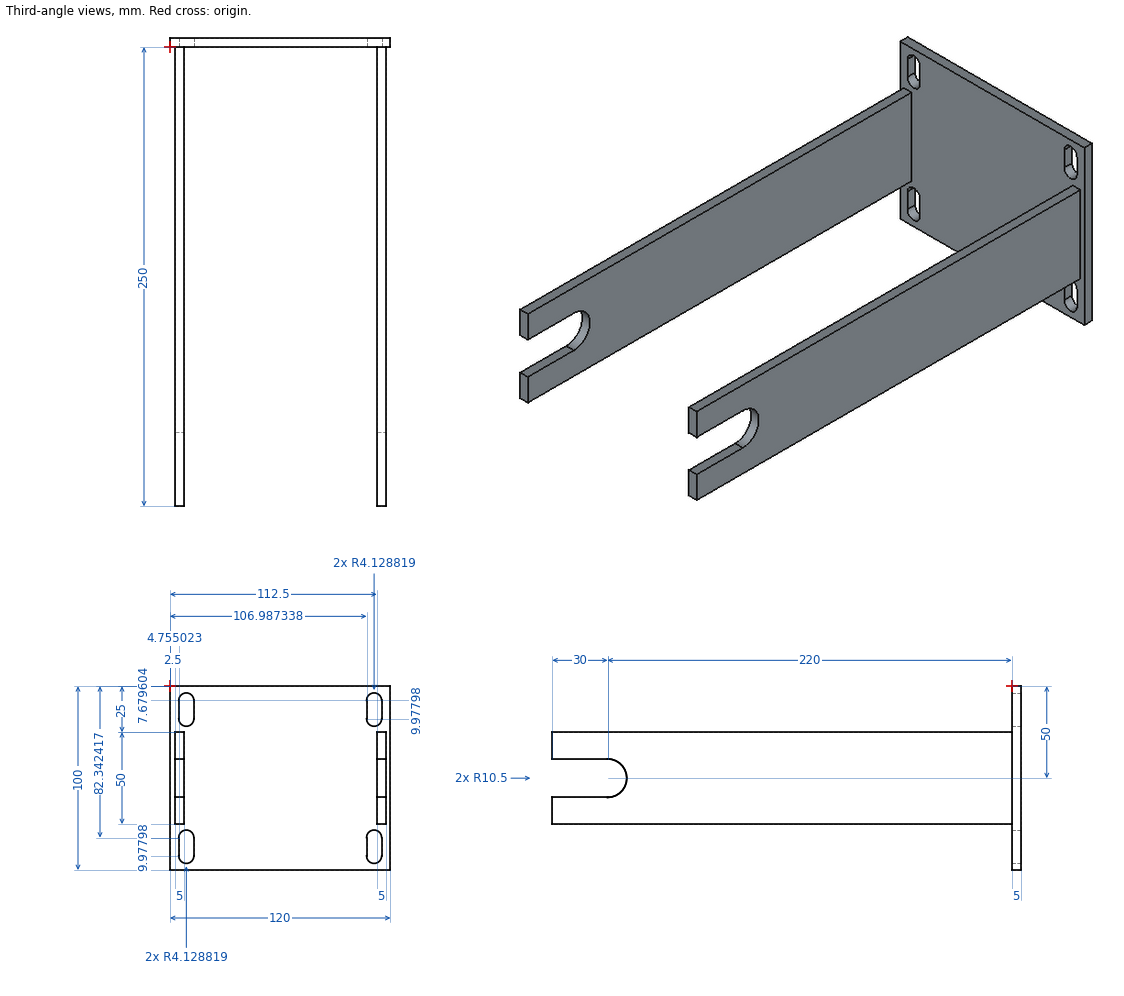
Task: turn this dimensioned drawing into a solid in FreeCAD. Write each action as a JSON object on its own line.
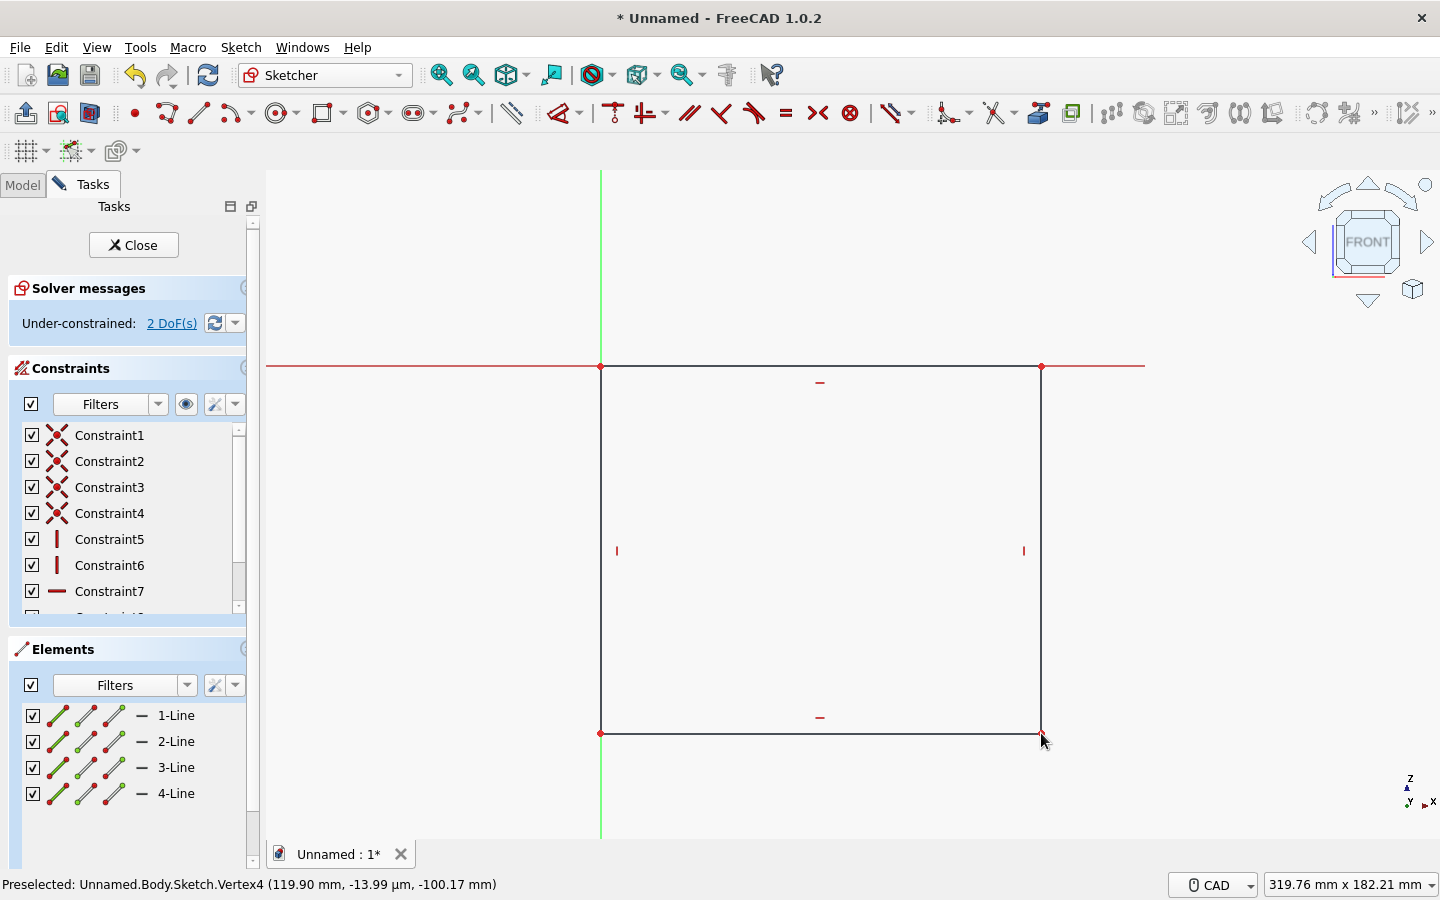
{"action": "left_click", "coordinate": [601, 477]}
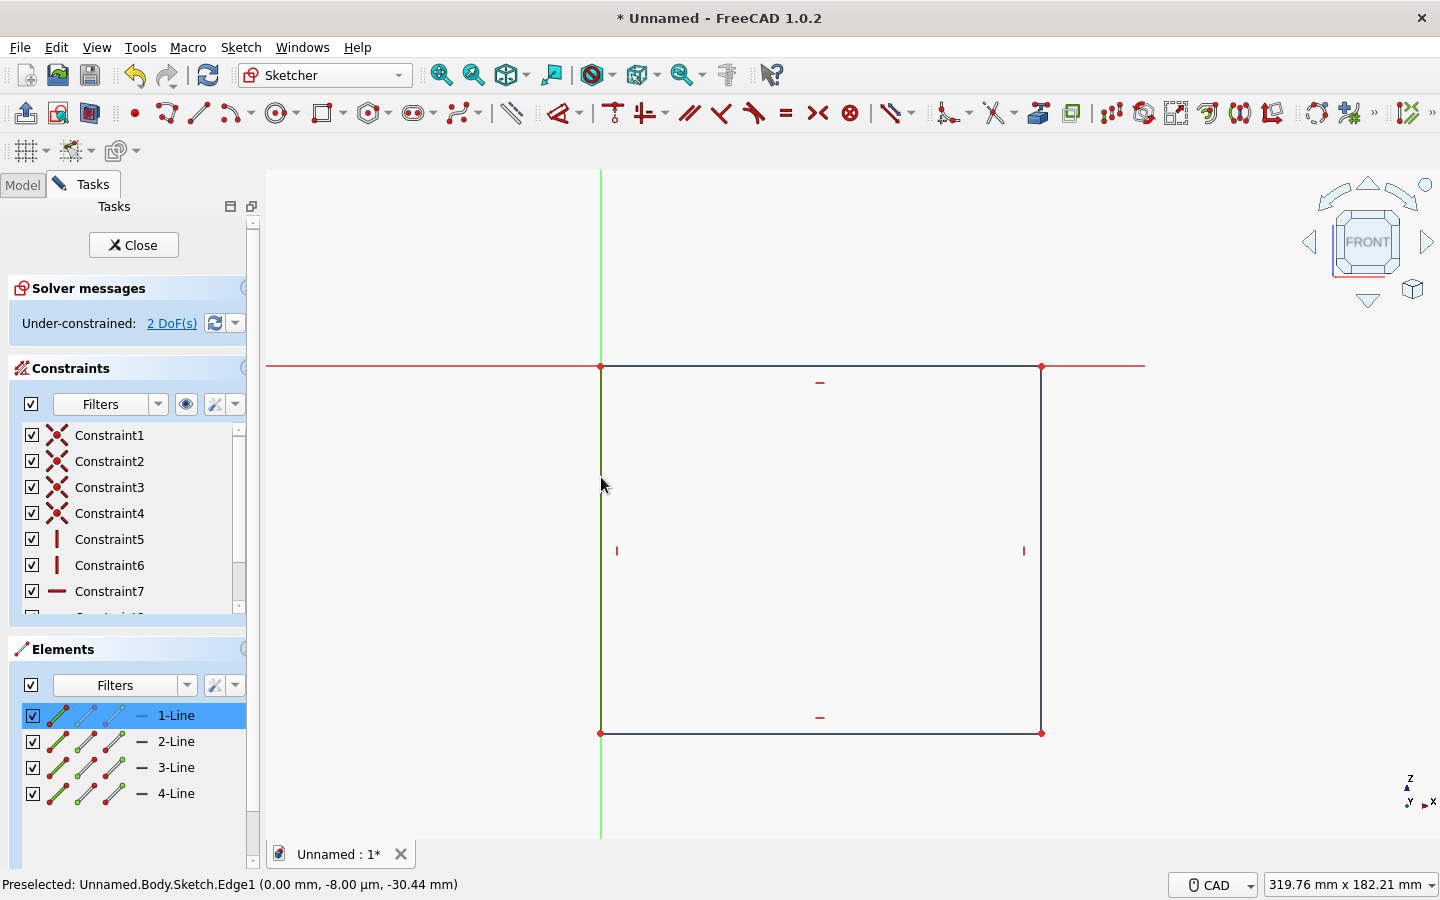
{"action": "left_click", "coordinate": [582, 114]}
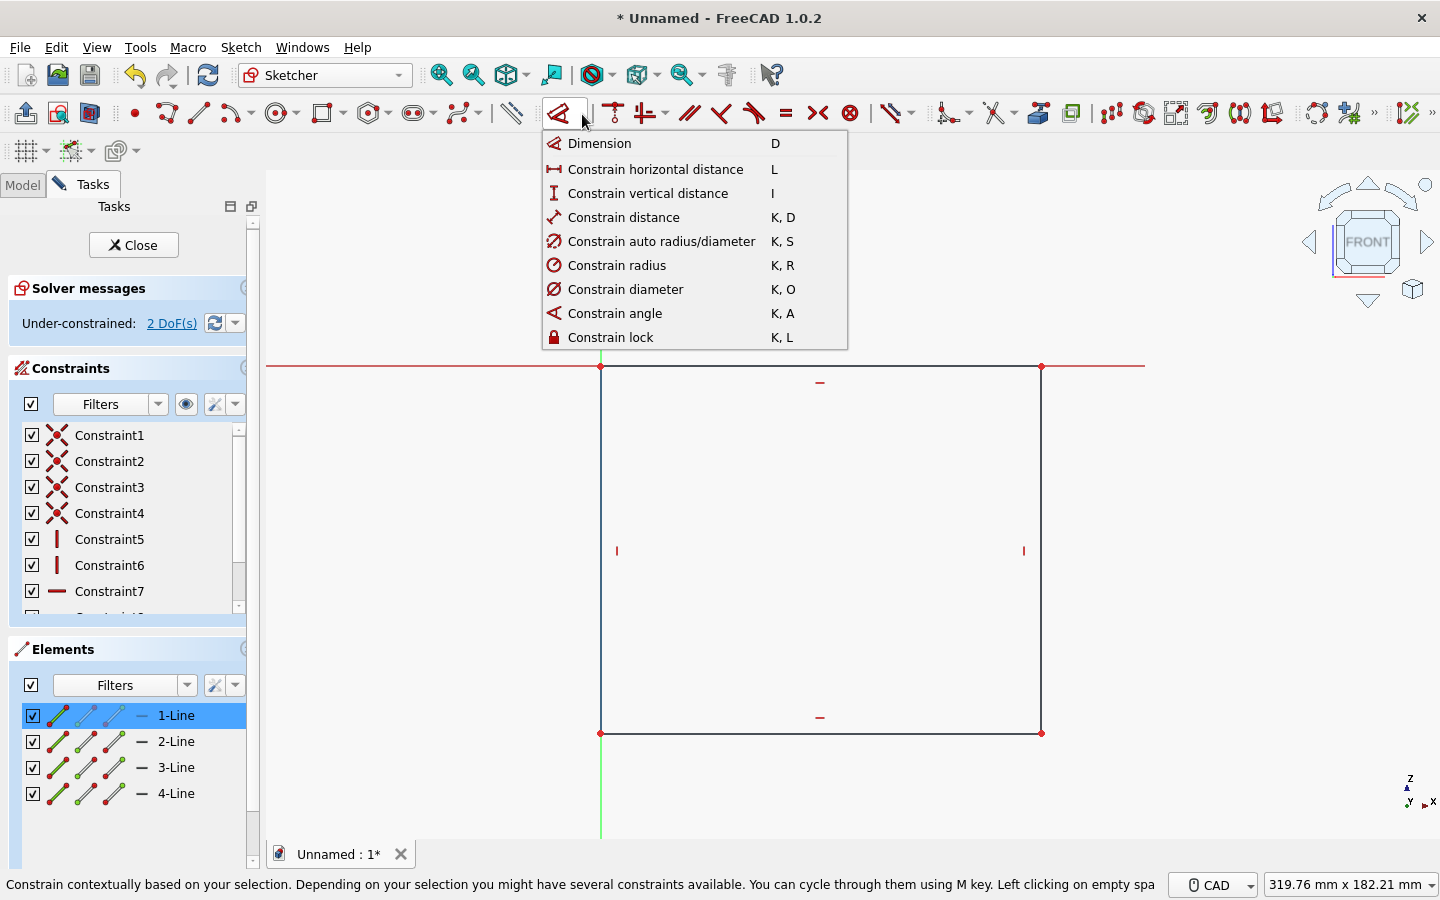
{"action": "left_click", "coordinate": [695, 193]}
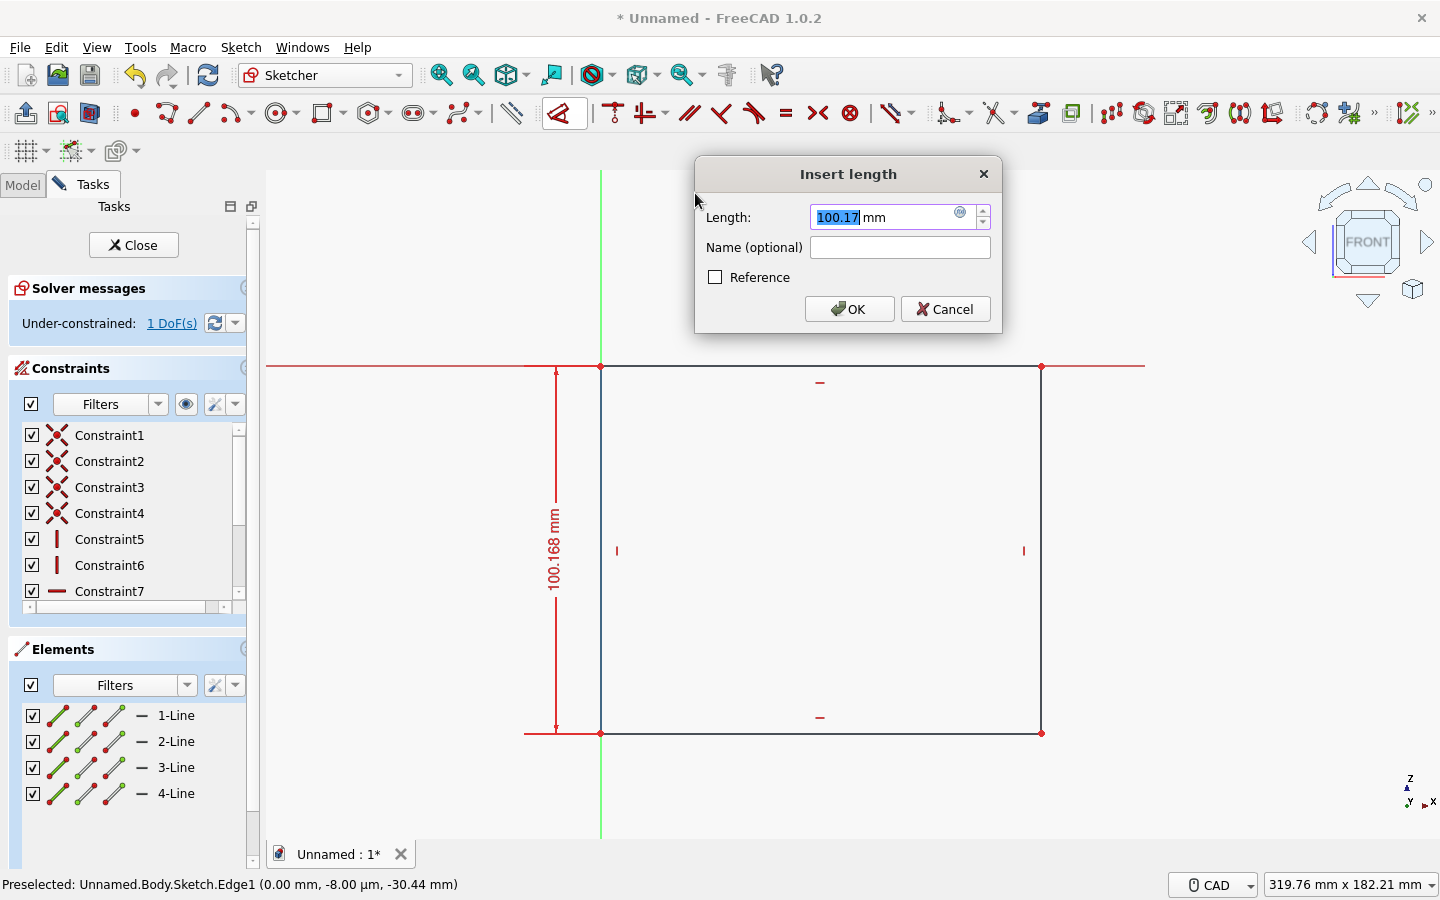
{"action": "type", "text": "100"}
{"action": "key", "text": "Return"}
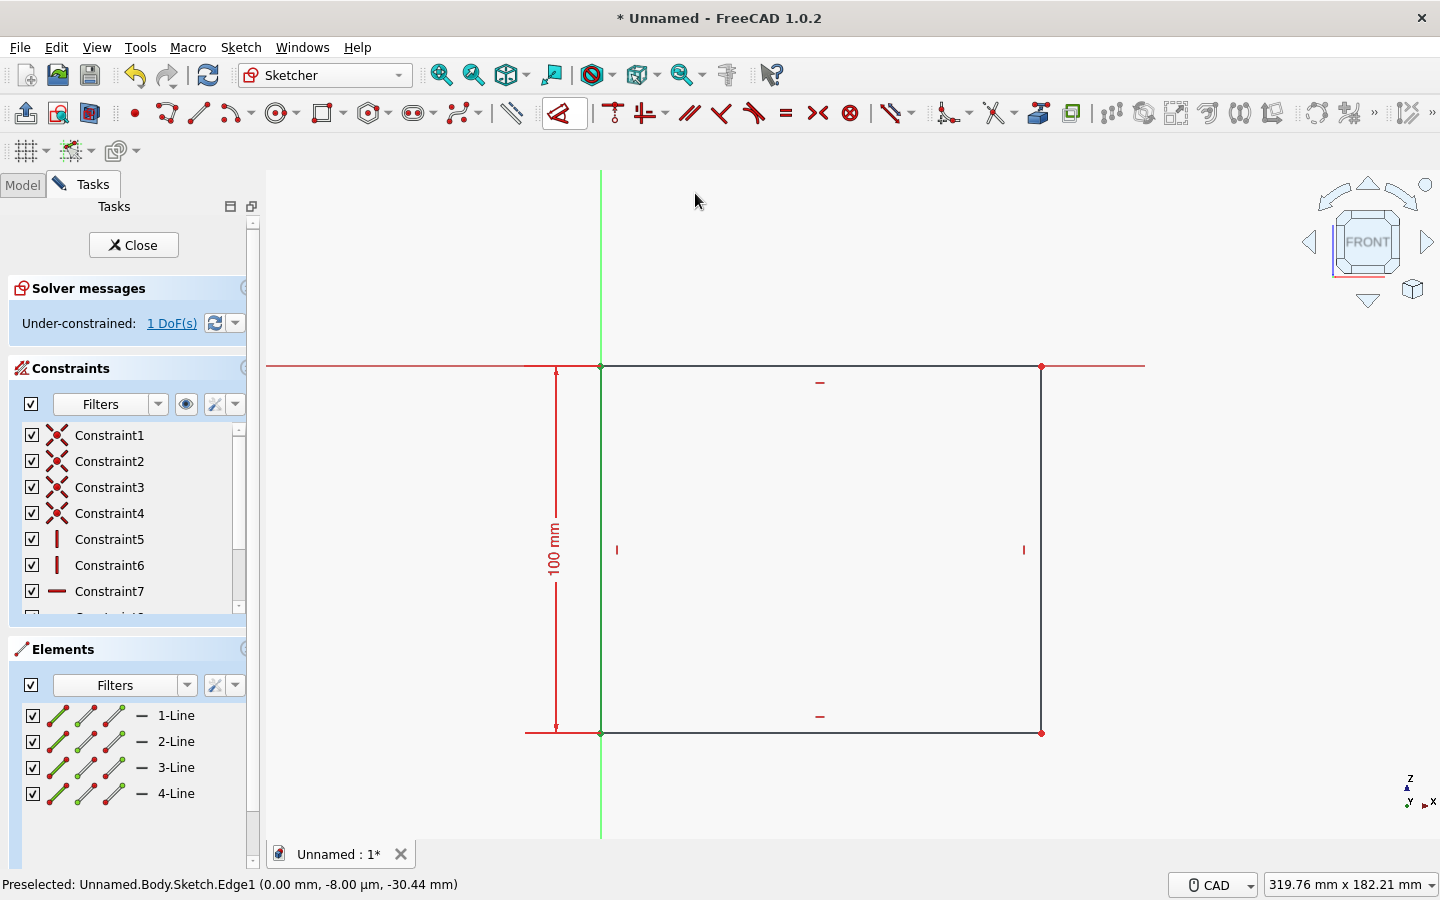
{"action": "left_click", "coordinate": [733, 733]}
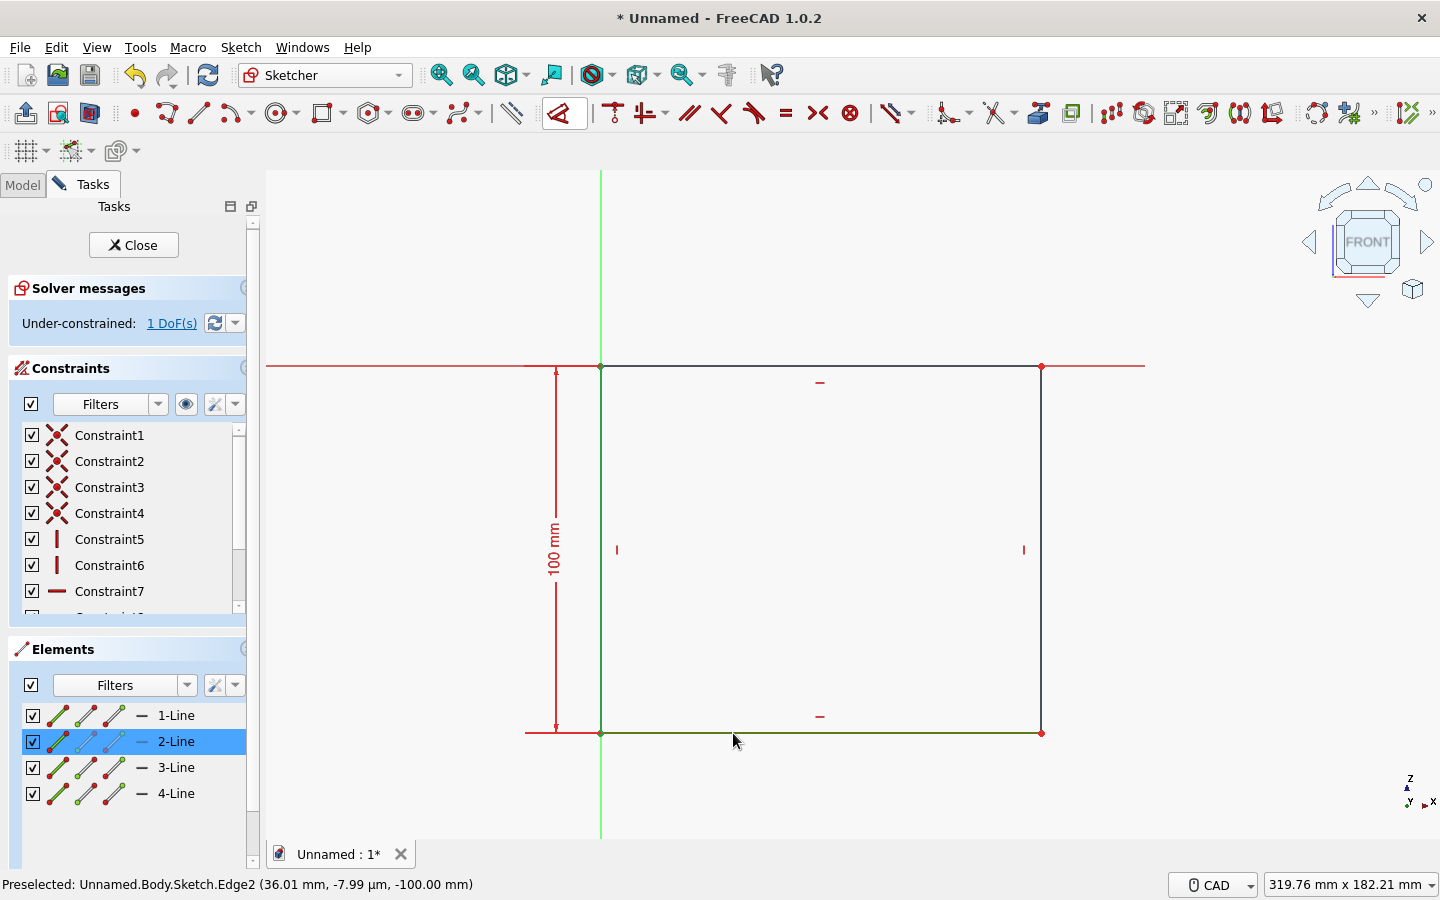
{"action": "key", "text": "l"}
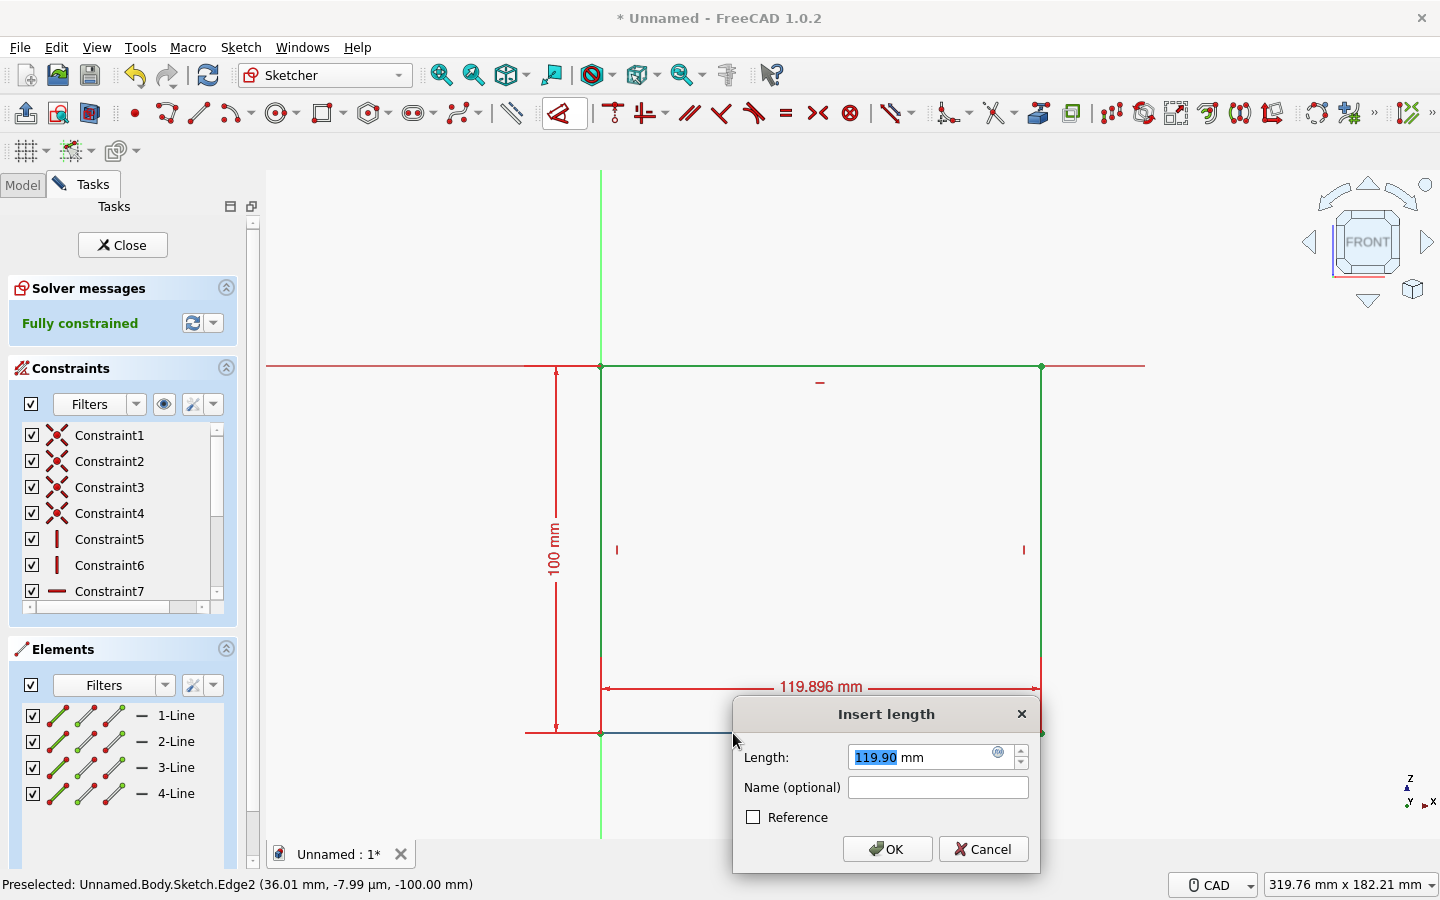
{"action": "type", "text": "120"}
{"action": "key", "text": "Return"}